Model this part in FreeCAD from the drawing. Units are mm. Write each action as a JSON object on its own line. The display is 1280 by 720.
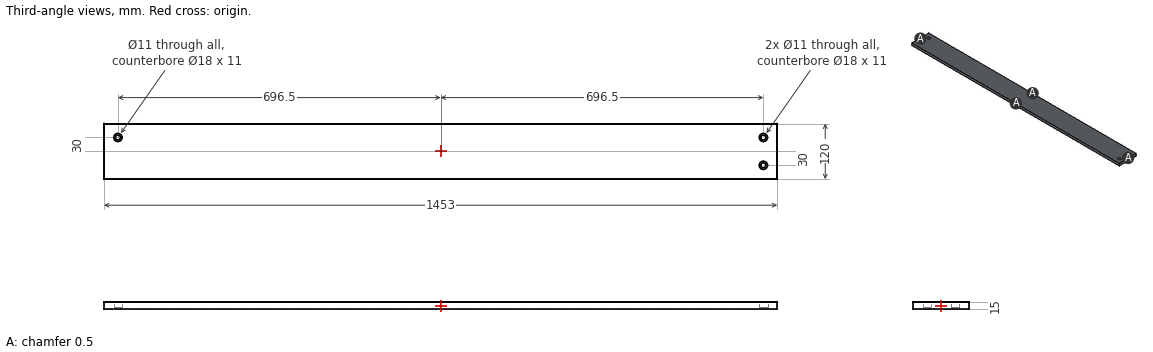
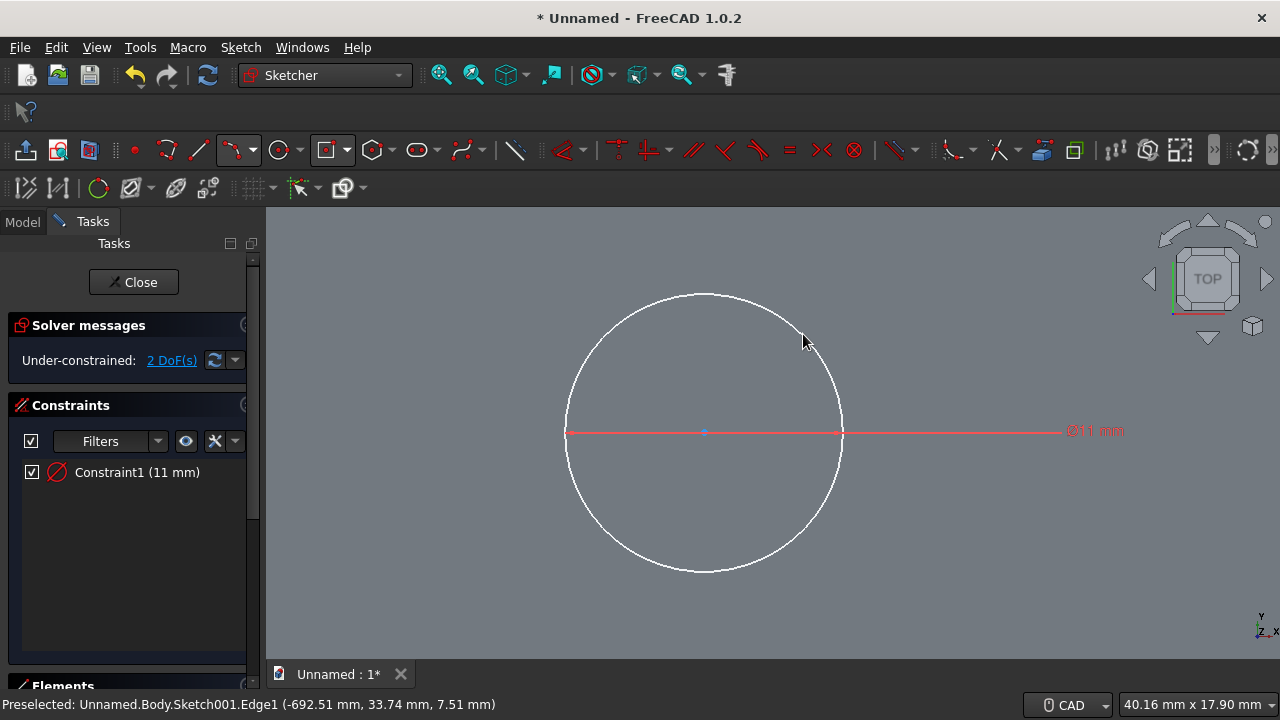
{"action": "left_click", "coordinate": [562, 150]}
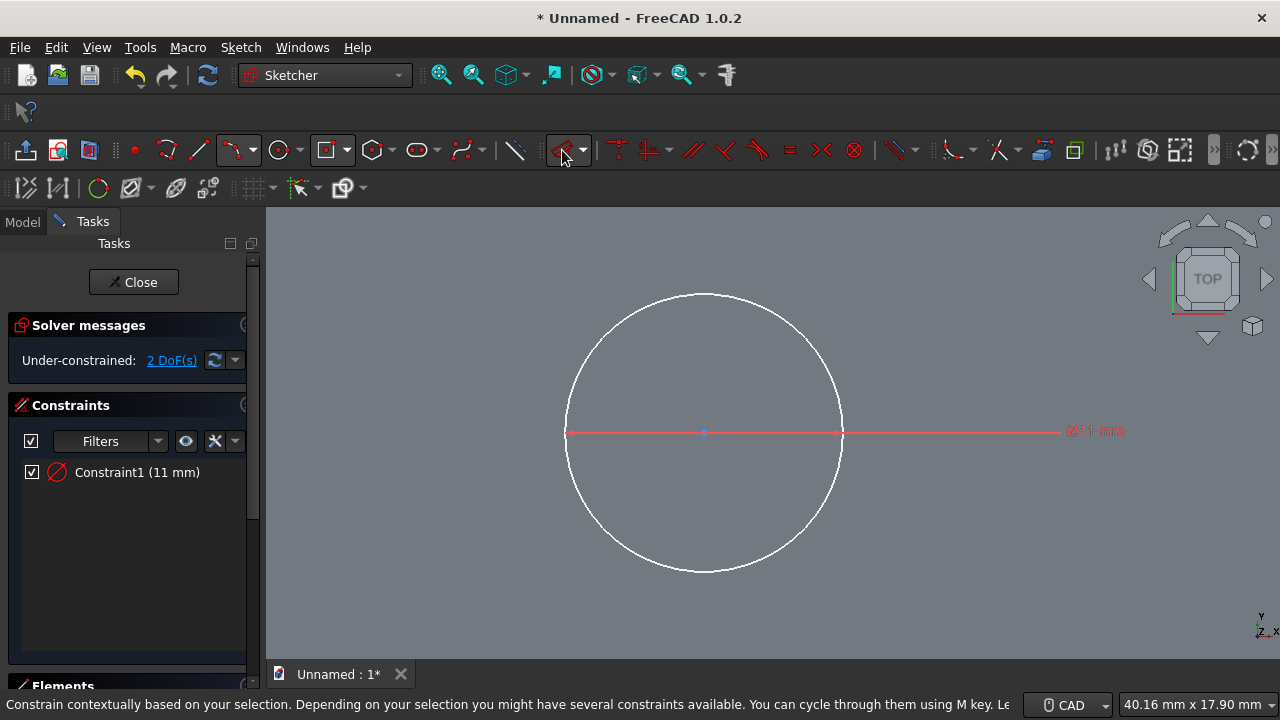
{"action": "left_click", "coordinate": [704, 433]}
{"action": "left_click", "coordinate": [670, 532]}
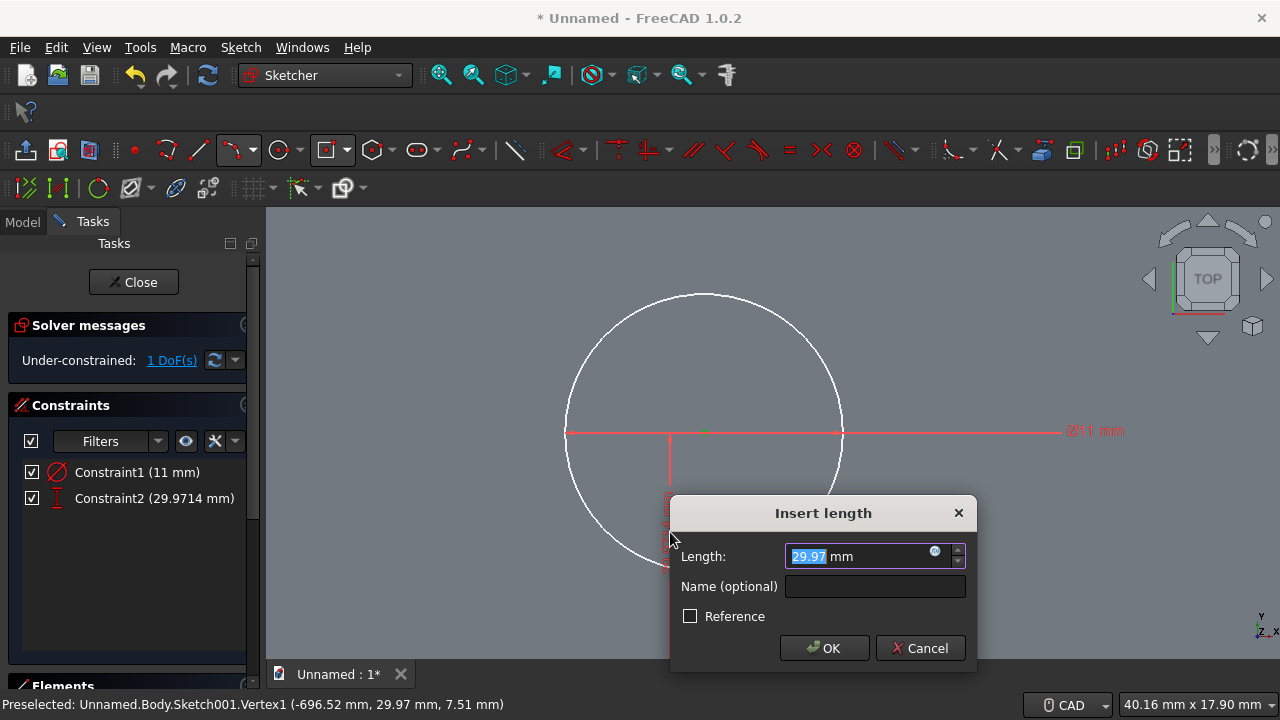
{"action": "type", "text": "30"}
{"action": "key", "text": "Return"}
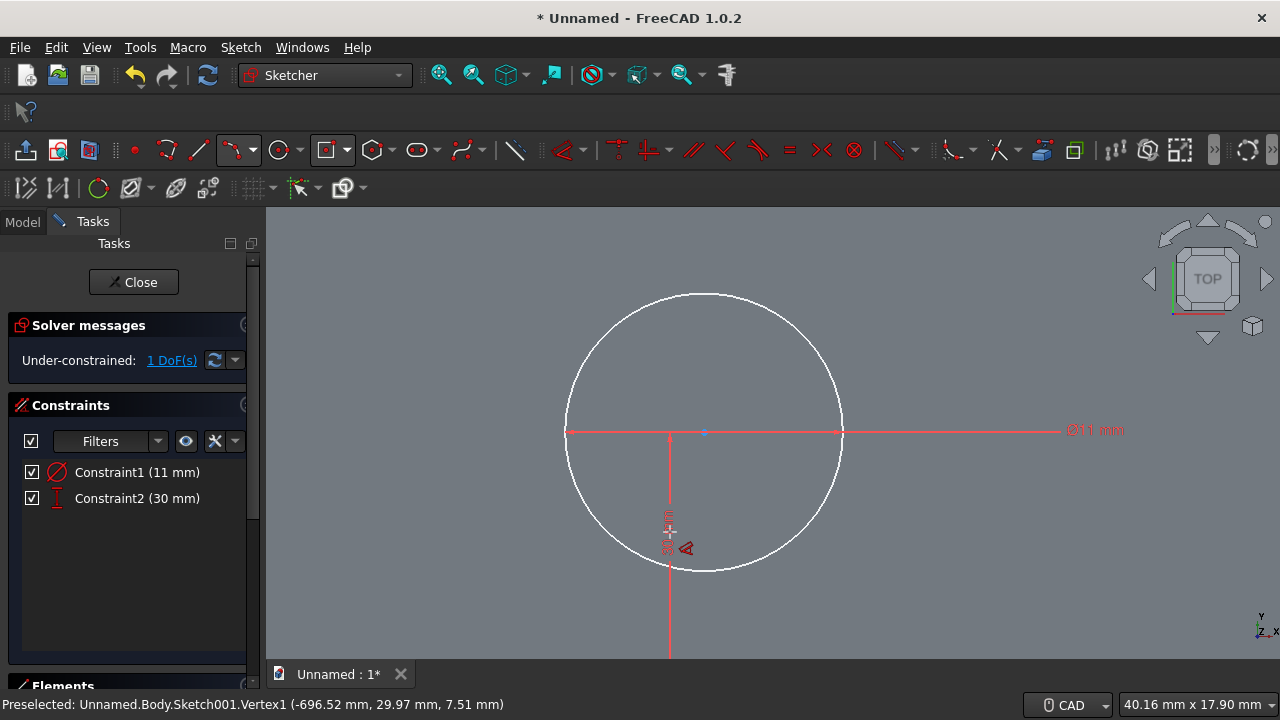
{"action": "left_click", "coordinate": [704, 432]}
{"action": "left_click", "coordinate": [910, 398]}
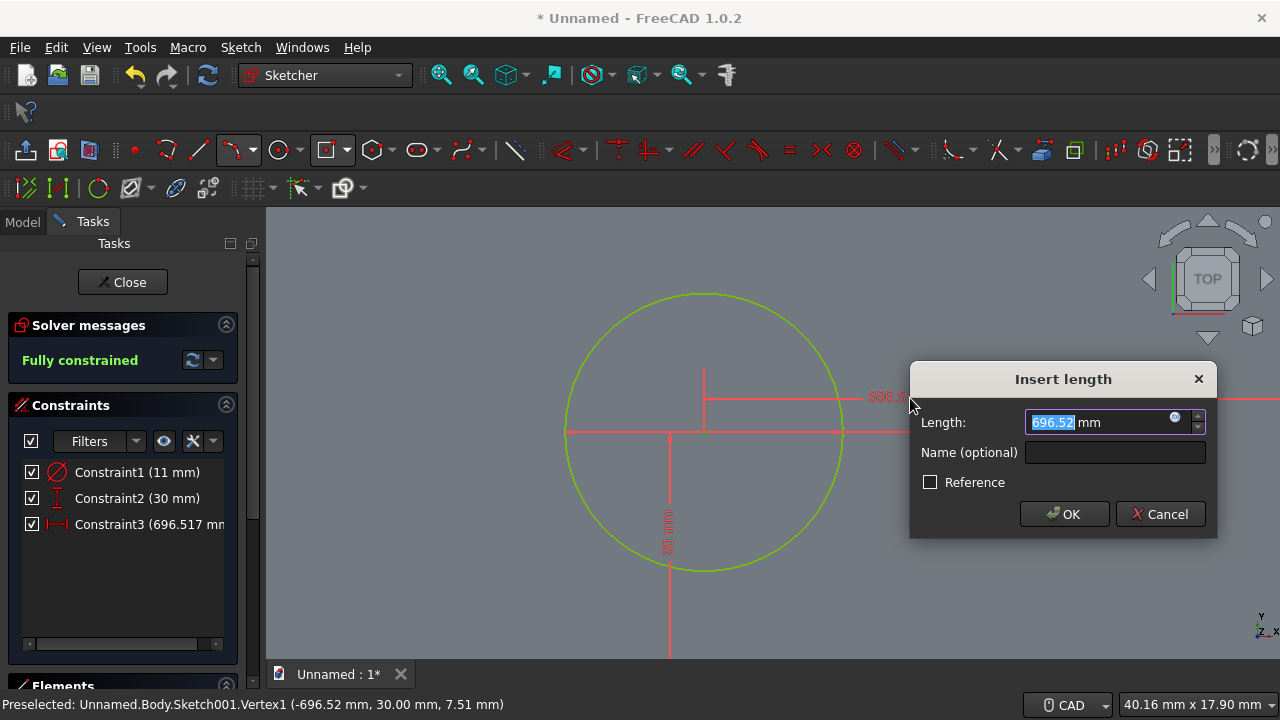
{"action": "type", "text": "696.5"}
{"action": "key", "text": "Return"}
{"action": "key", "text": "Escape"}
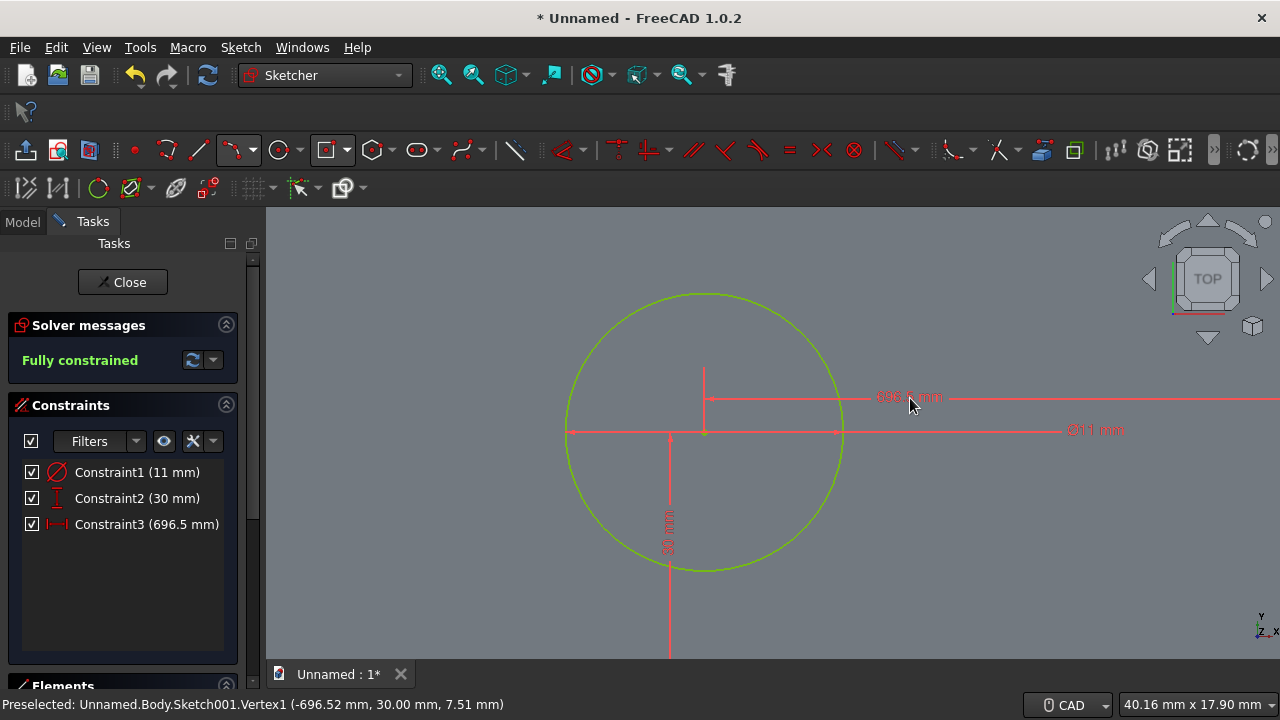
{"action": "left_click", "coordinate": [123, 282]}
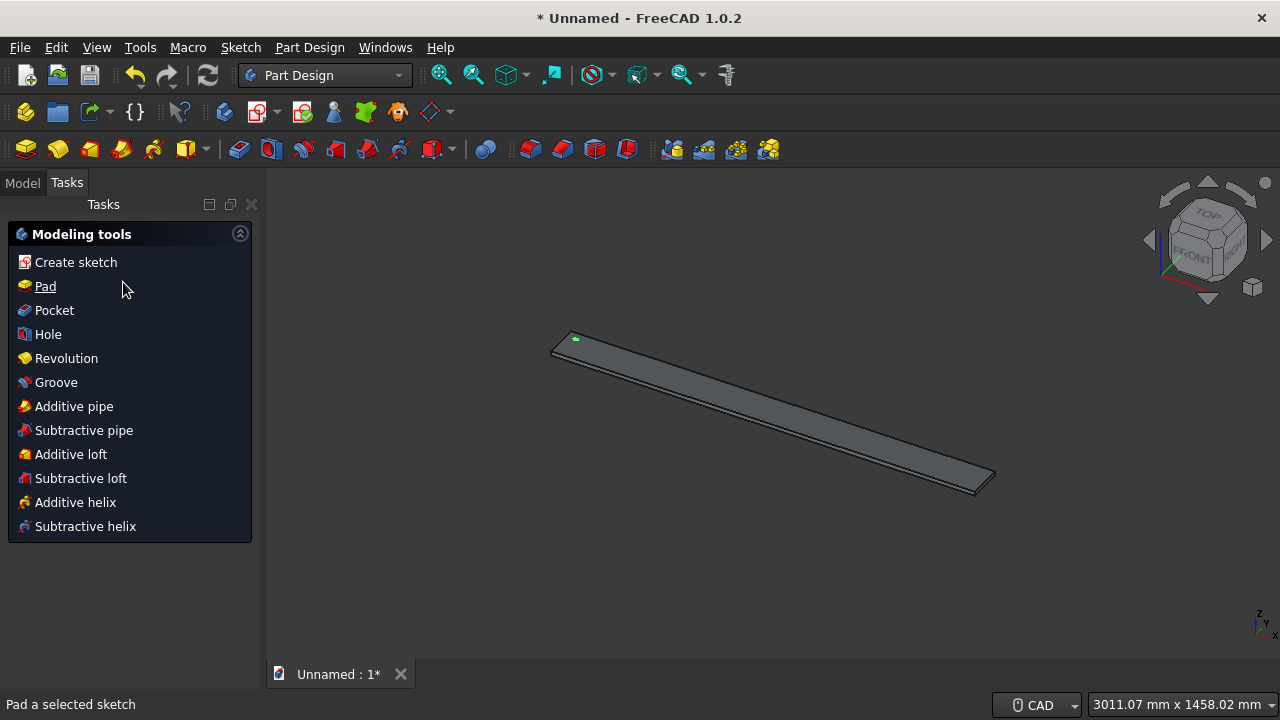
{"action": "left_click", "coordinate": [272, 150]}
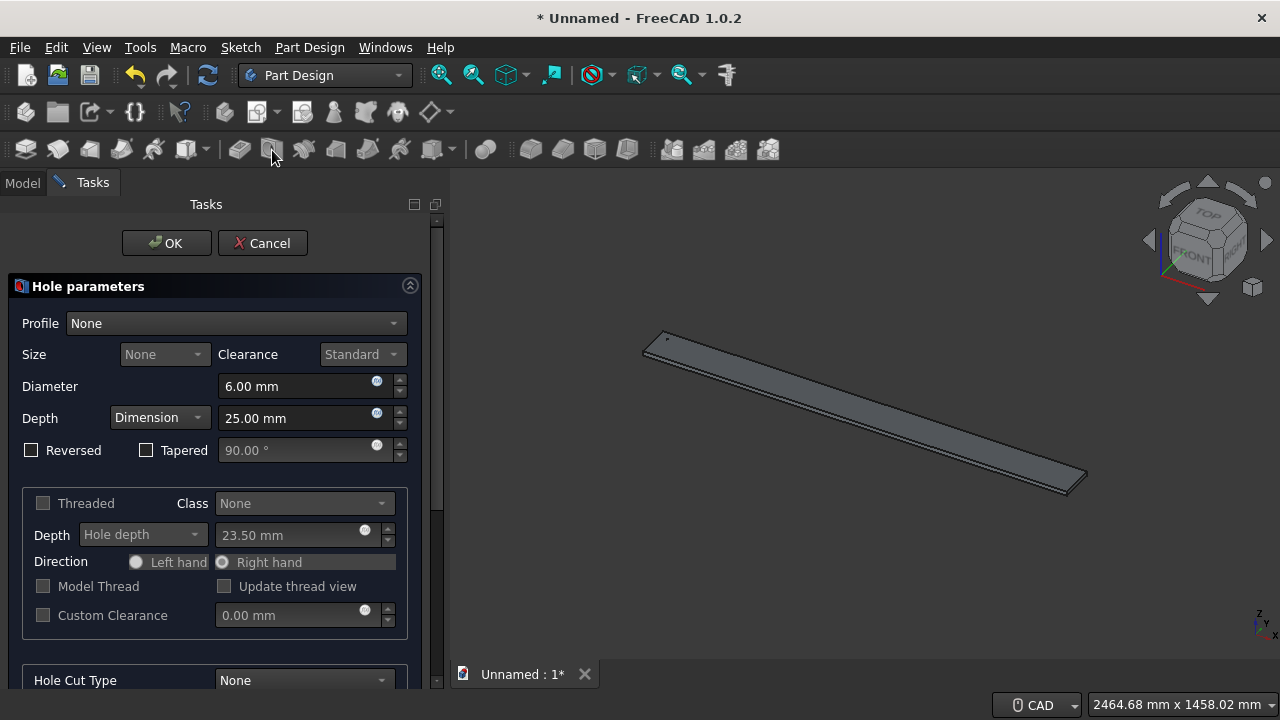
{"action": "triple_click", "coordinate": [305, 386]}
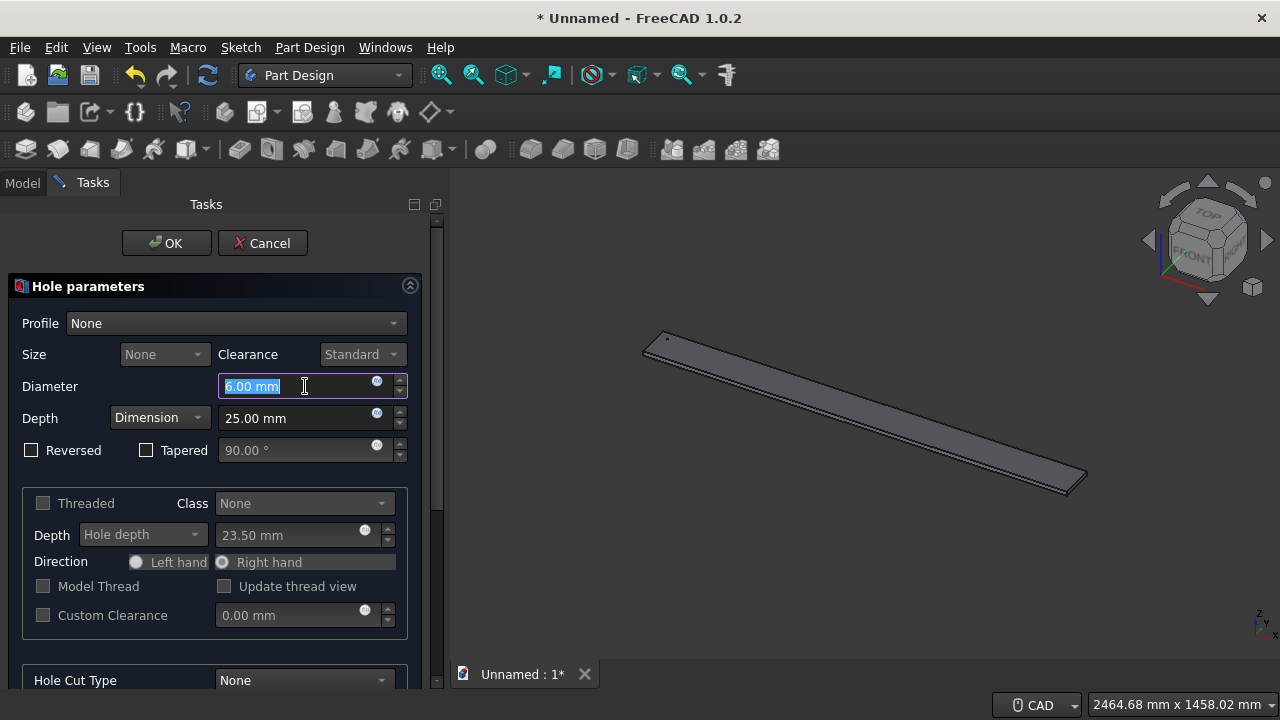
{"action": "type", "text": "11"}
{"action": "key", "text": "Tab"}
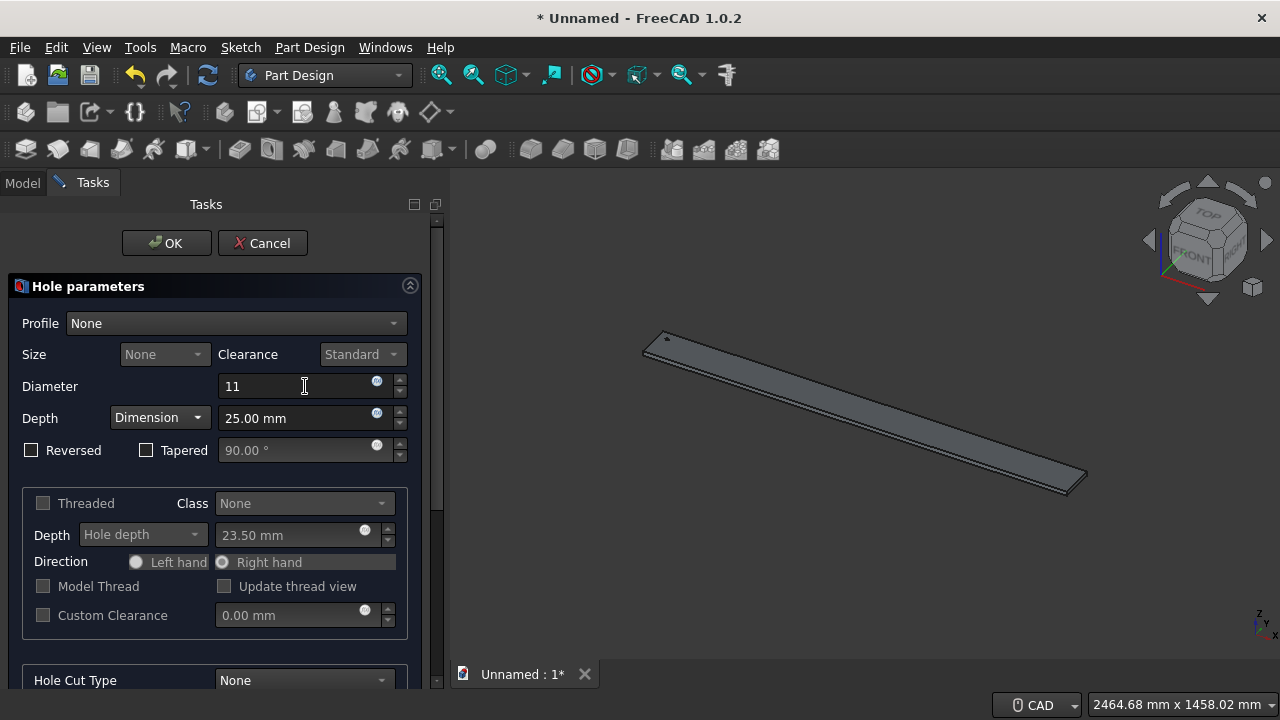
{"action": "left_click", "coordinate": [161, 418]}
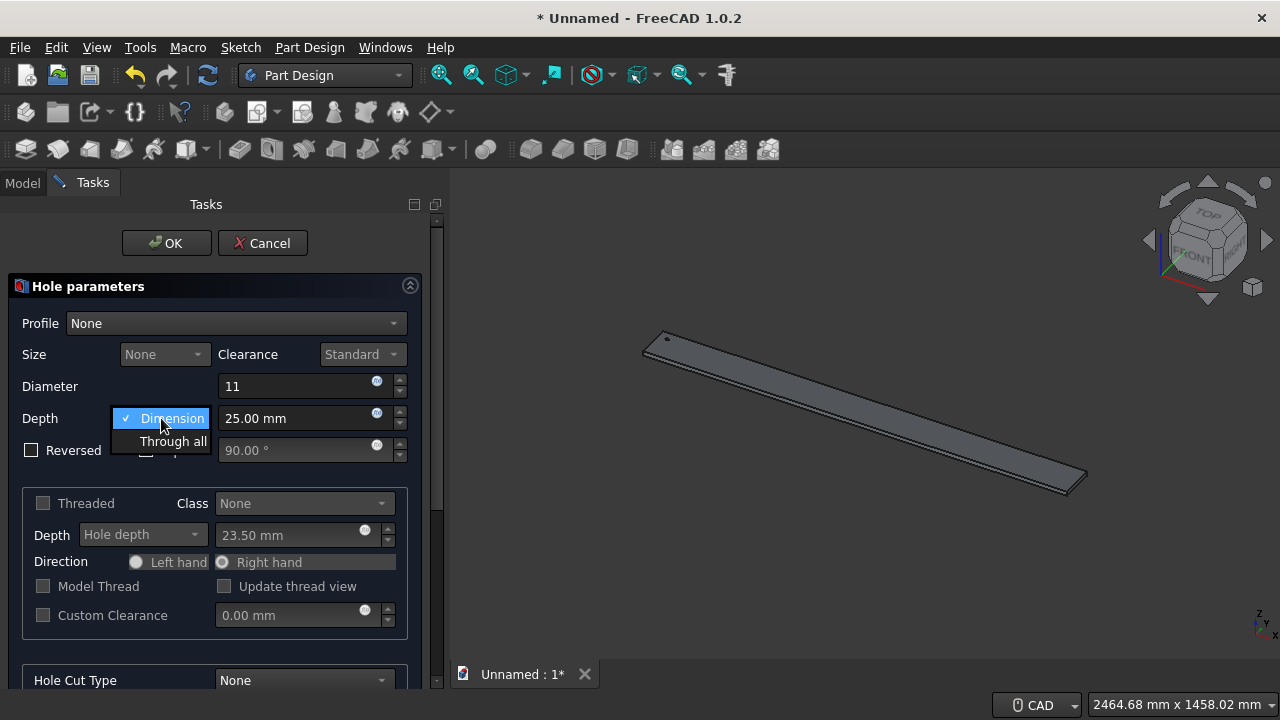
{"action": "left_click", "coordinate": [160, 442]}